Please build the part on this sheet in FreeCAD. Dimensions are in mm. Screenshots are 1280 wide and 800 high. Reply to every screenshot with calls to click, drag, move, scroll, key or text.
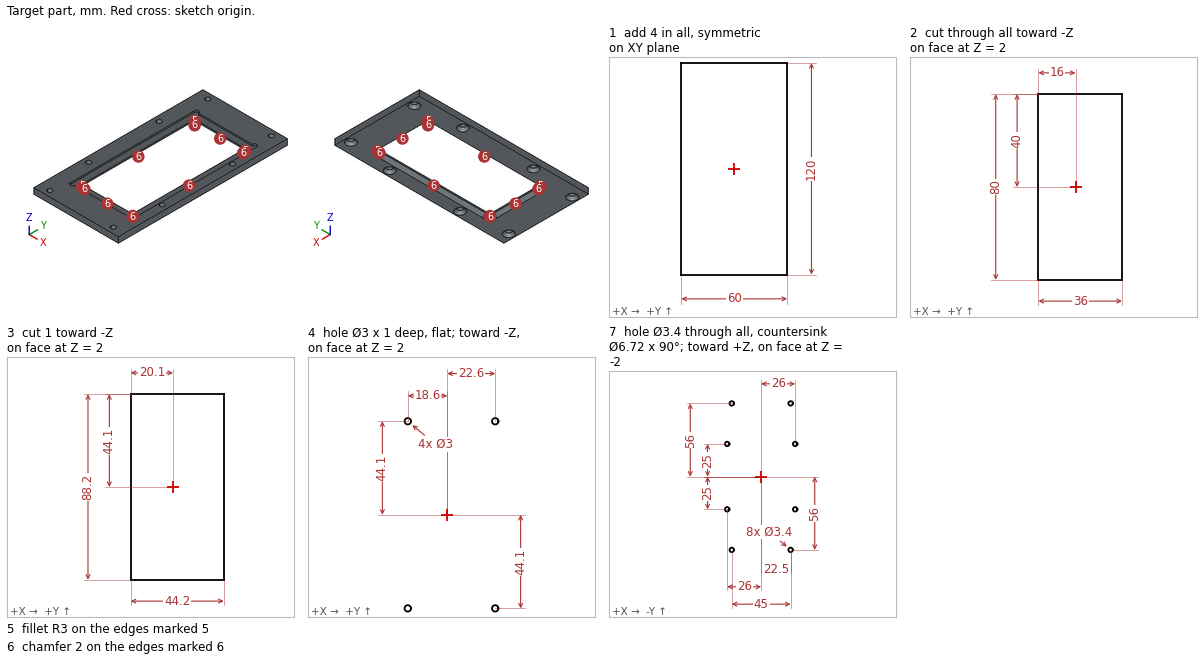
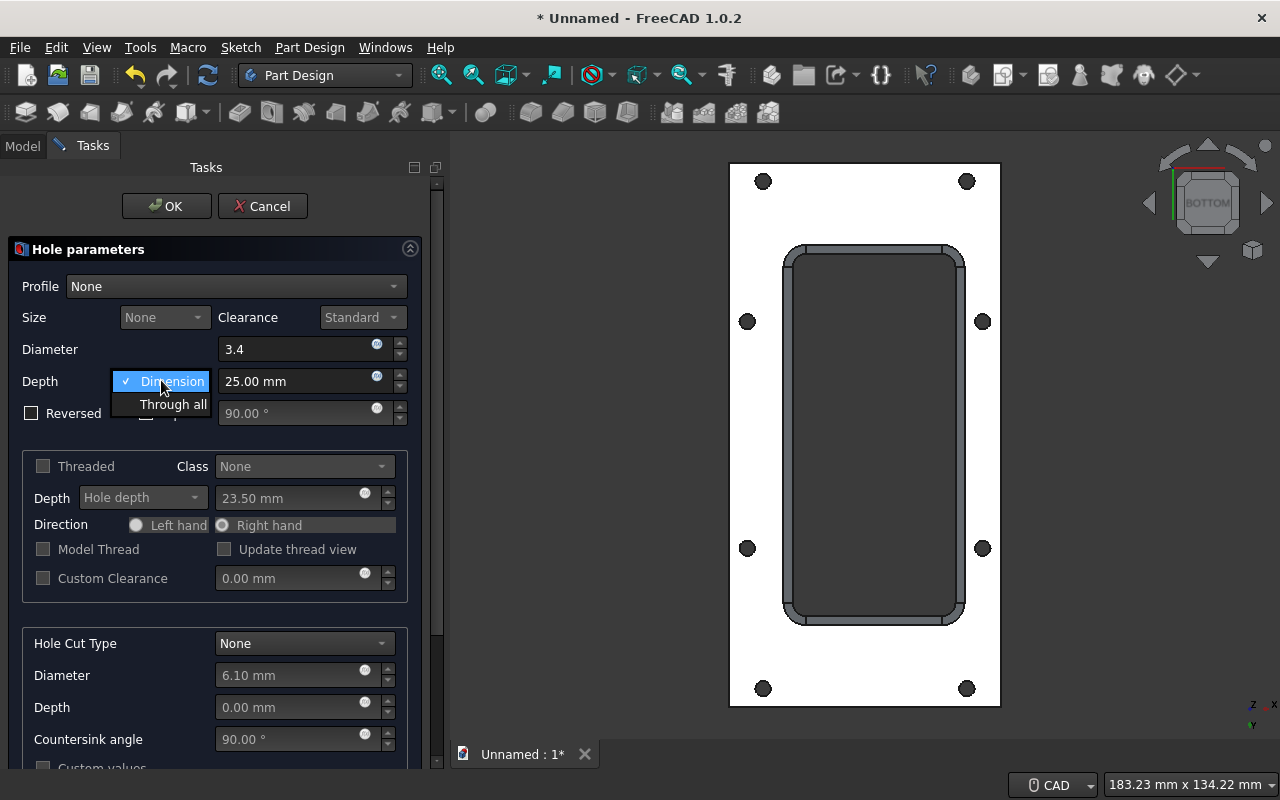
click(160, 404)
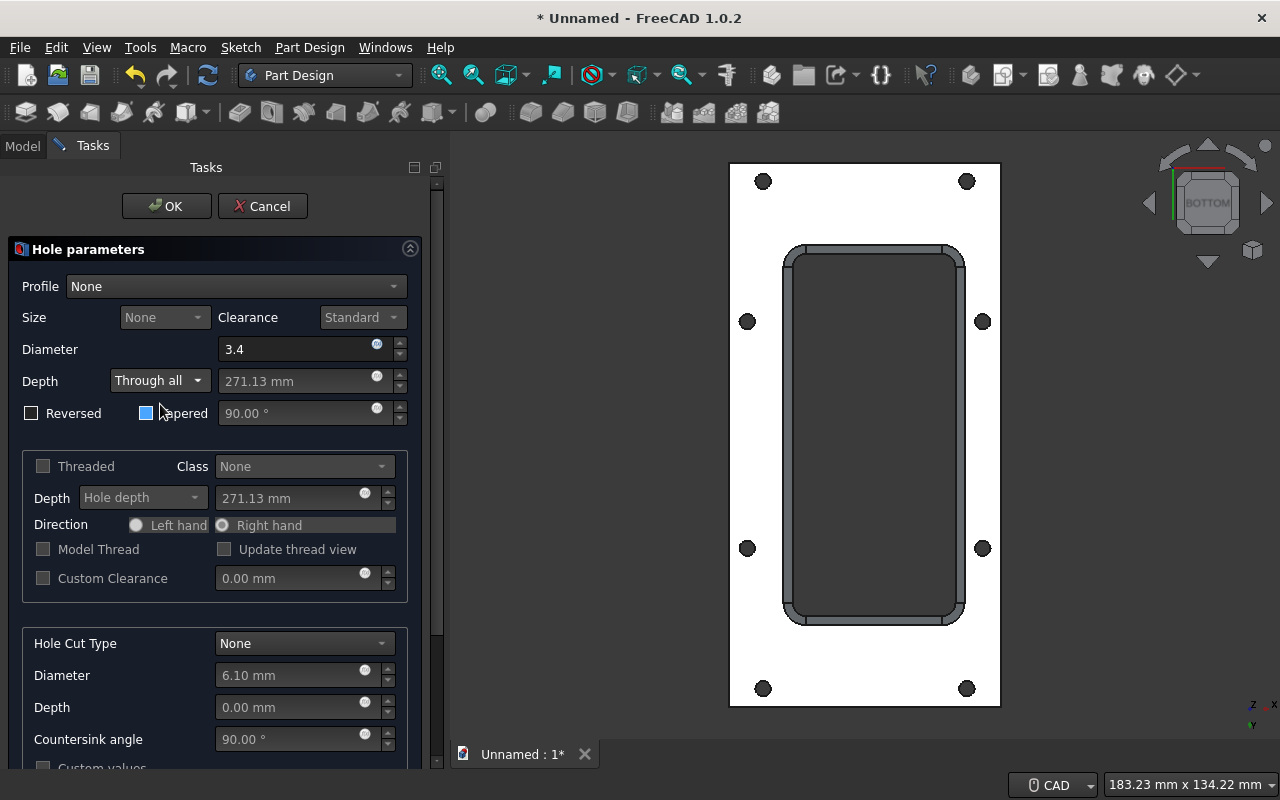
click(306, 644)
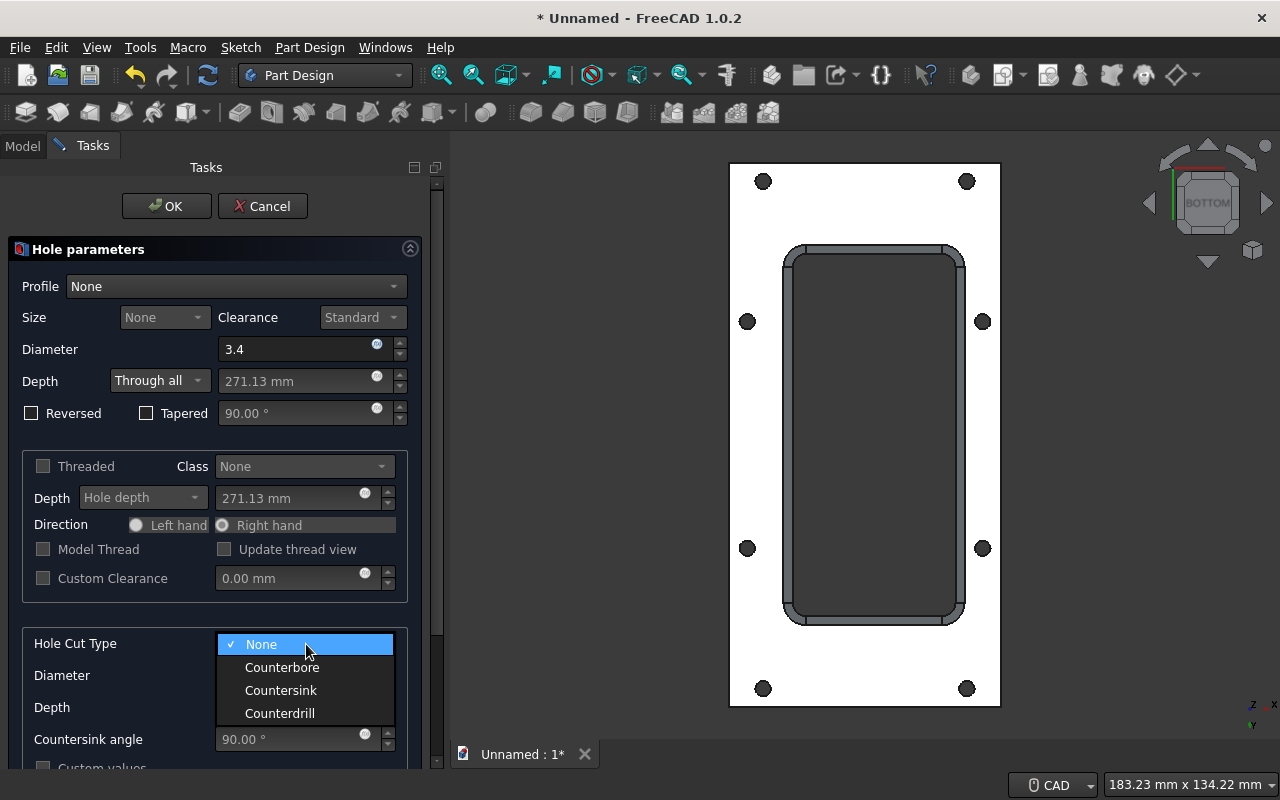
click(304, 690)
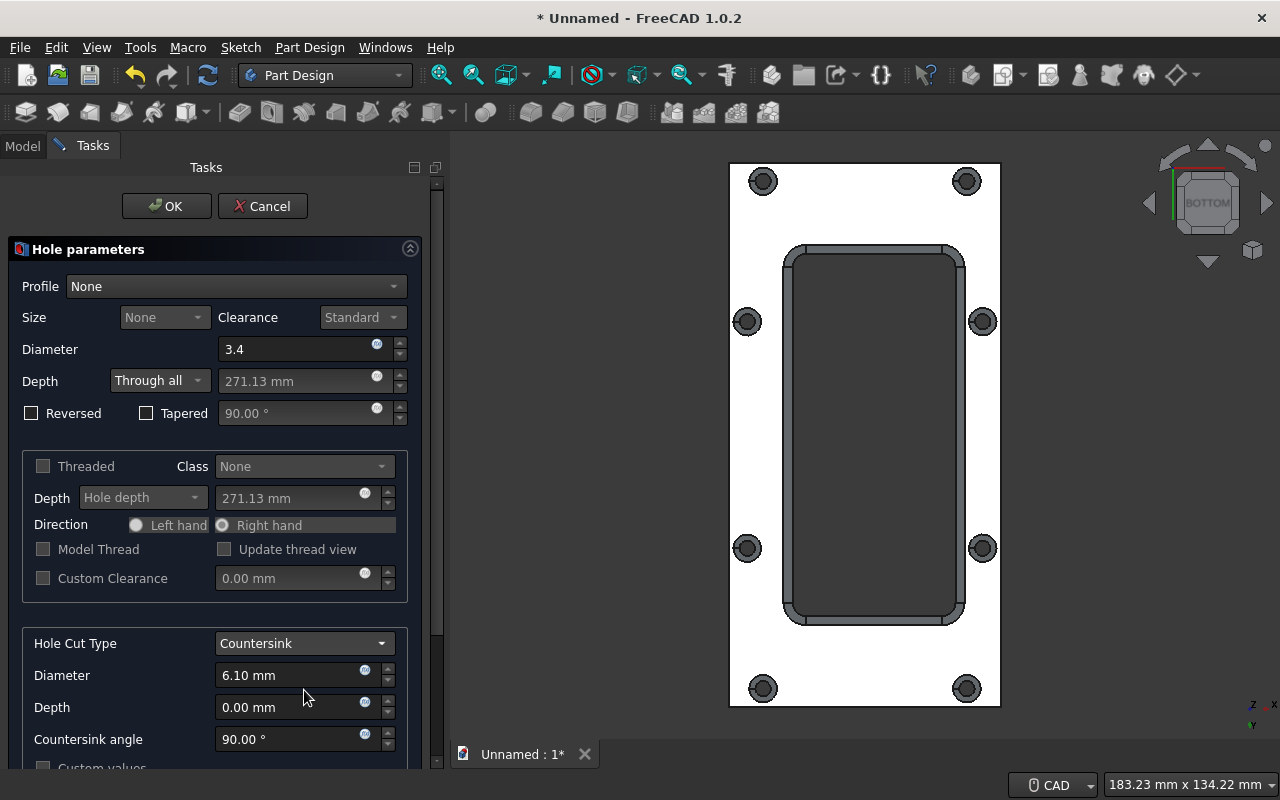
triple_click(298, 675)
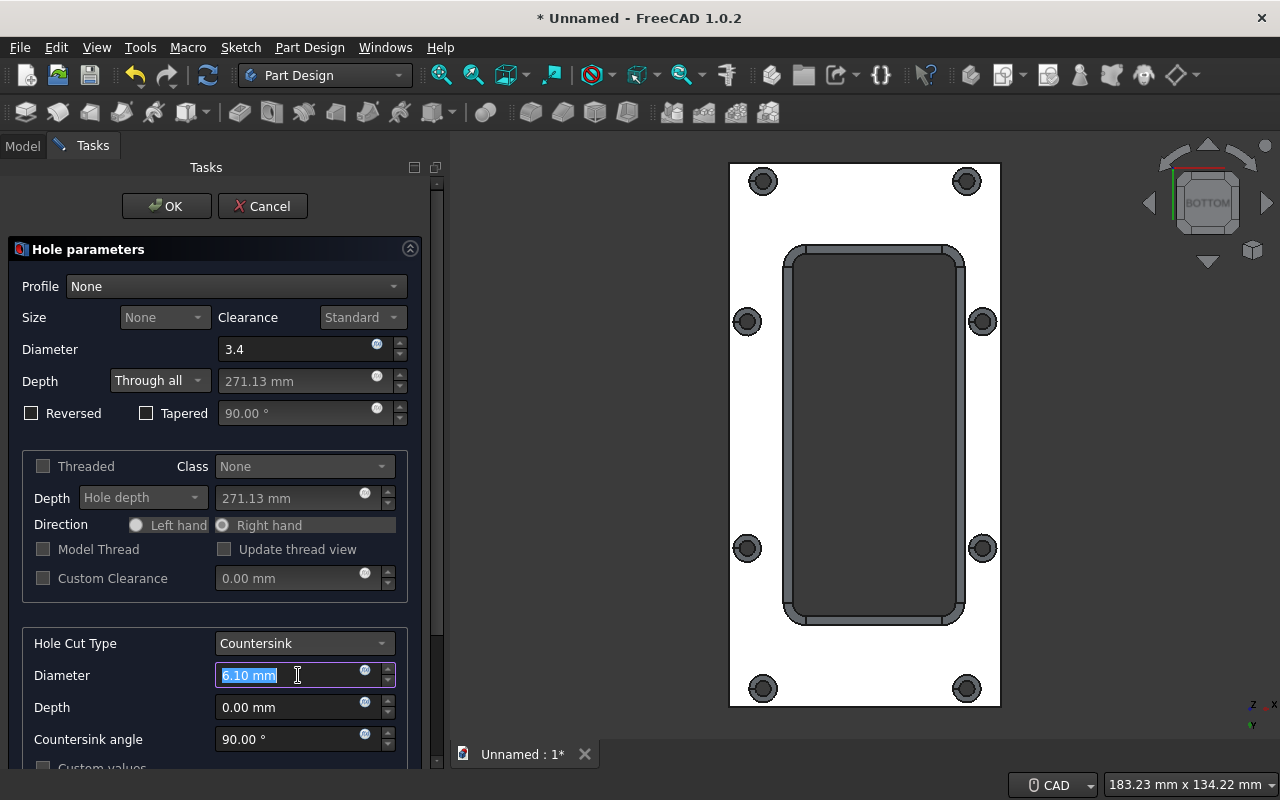
text(6.72)
key(Tab)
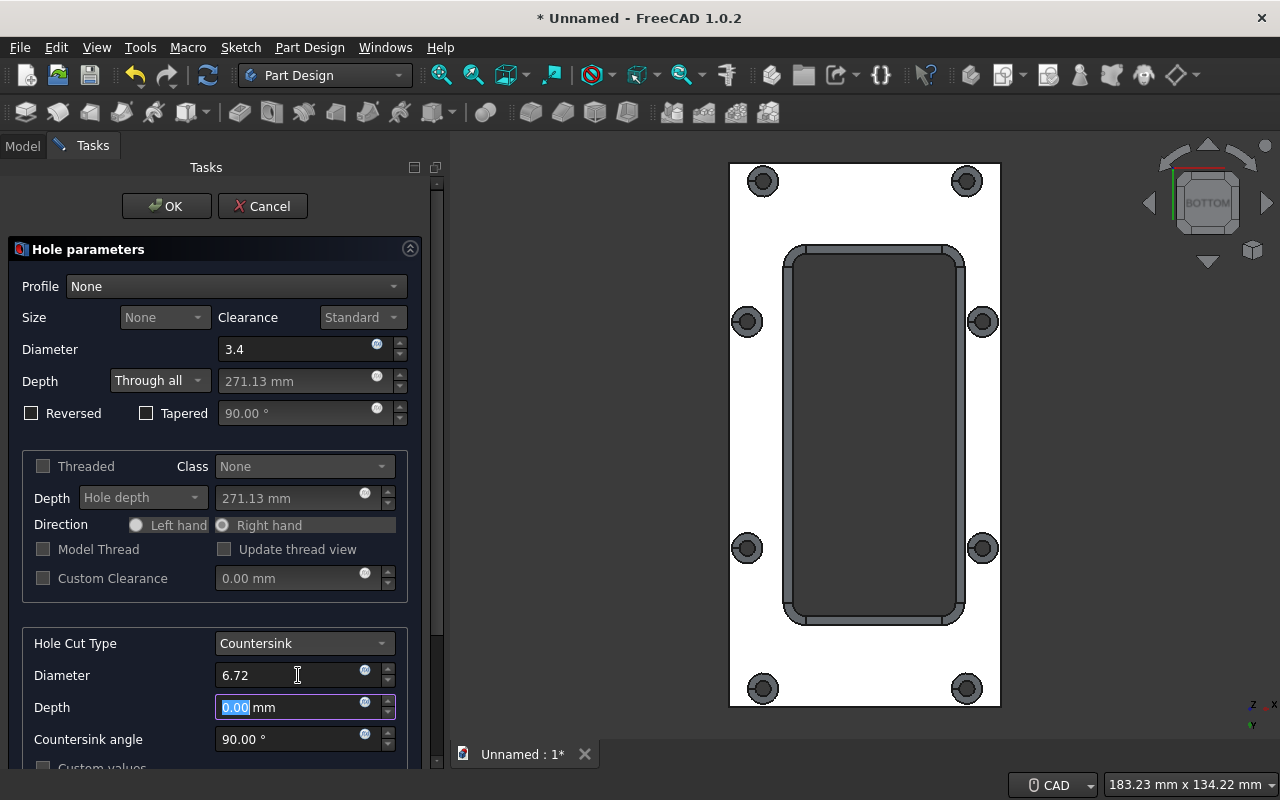
click(167, 206)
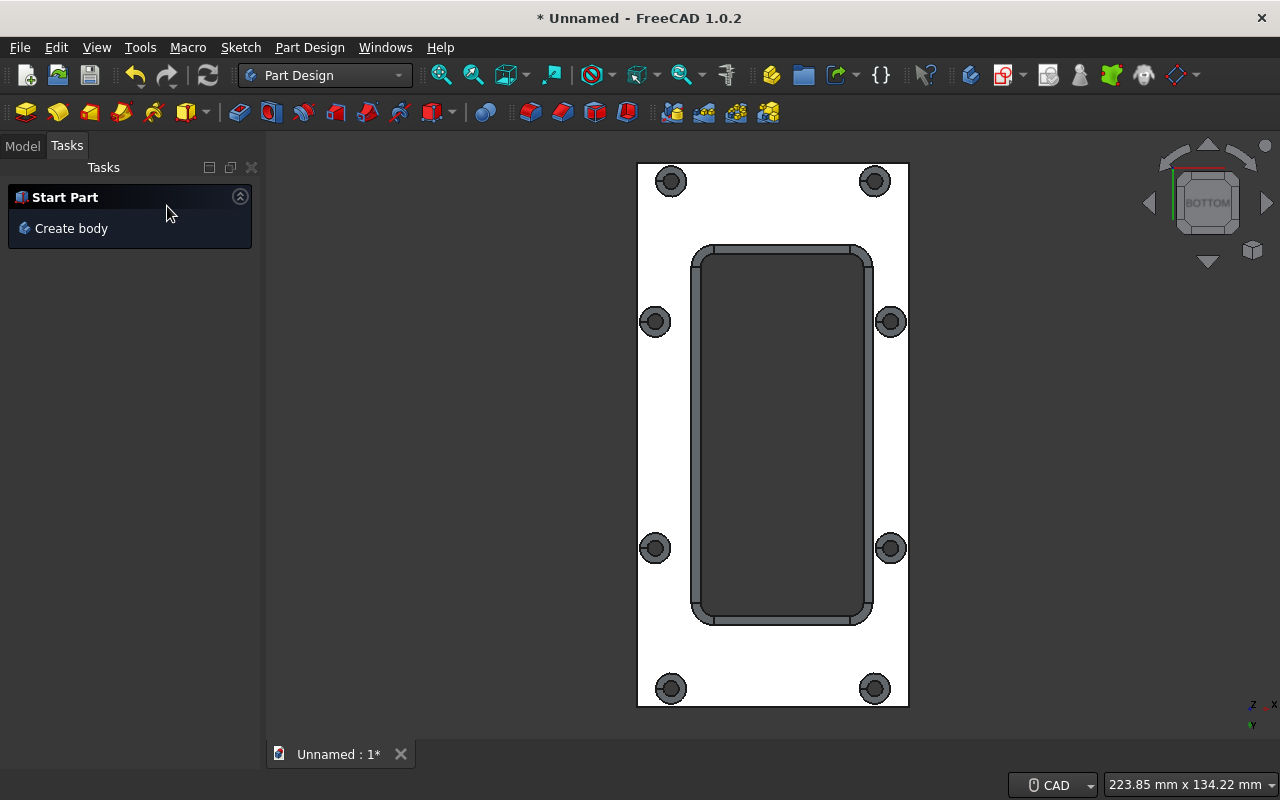
key(0)